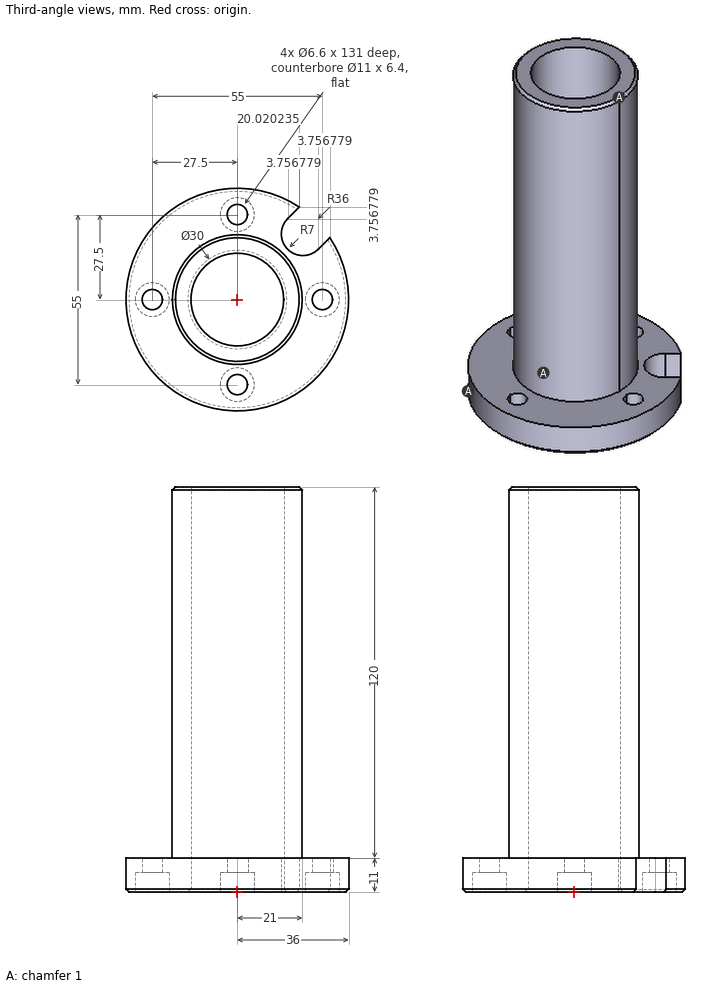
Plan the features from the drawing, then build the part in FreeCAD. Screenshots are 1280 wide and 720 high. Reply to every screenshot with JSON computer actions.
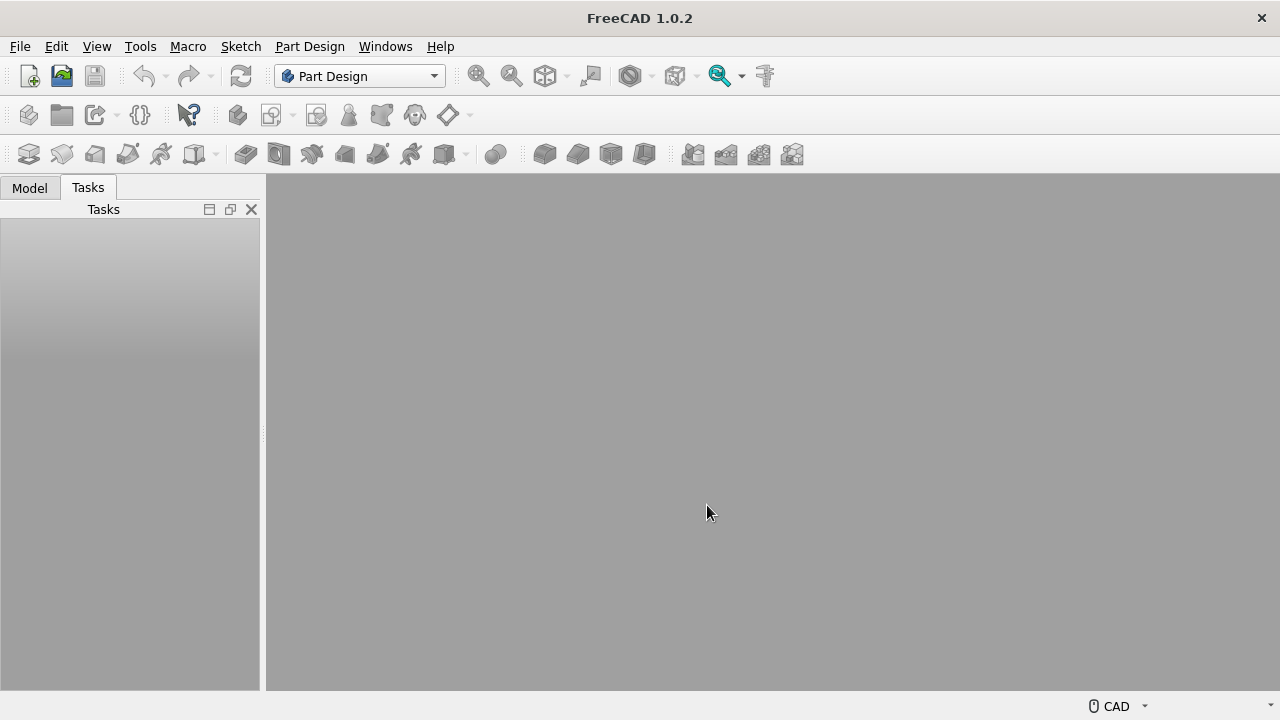
{"action": "left_click", "coordinate": [29, 76]}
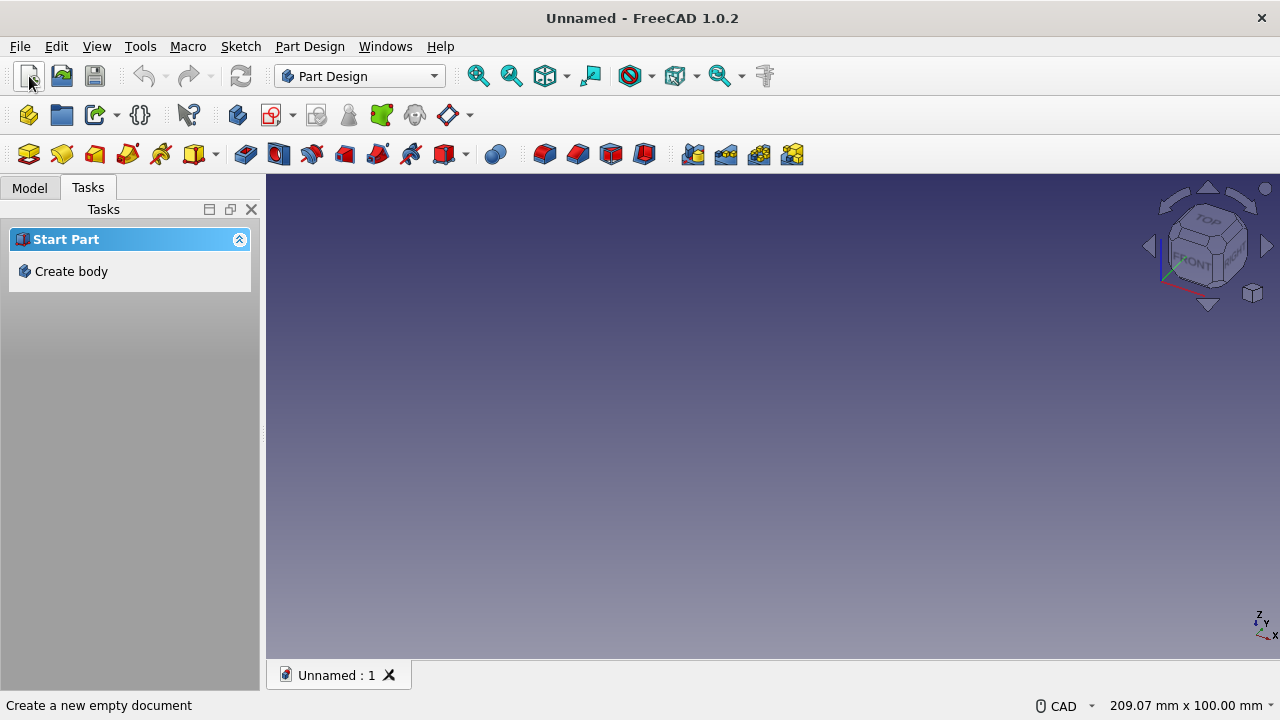
{"action": "left_click", "coordinate": [270, 116]}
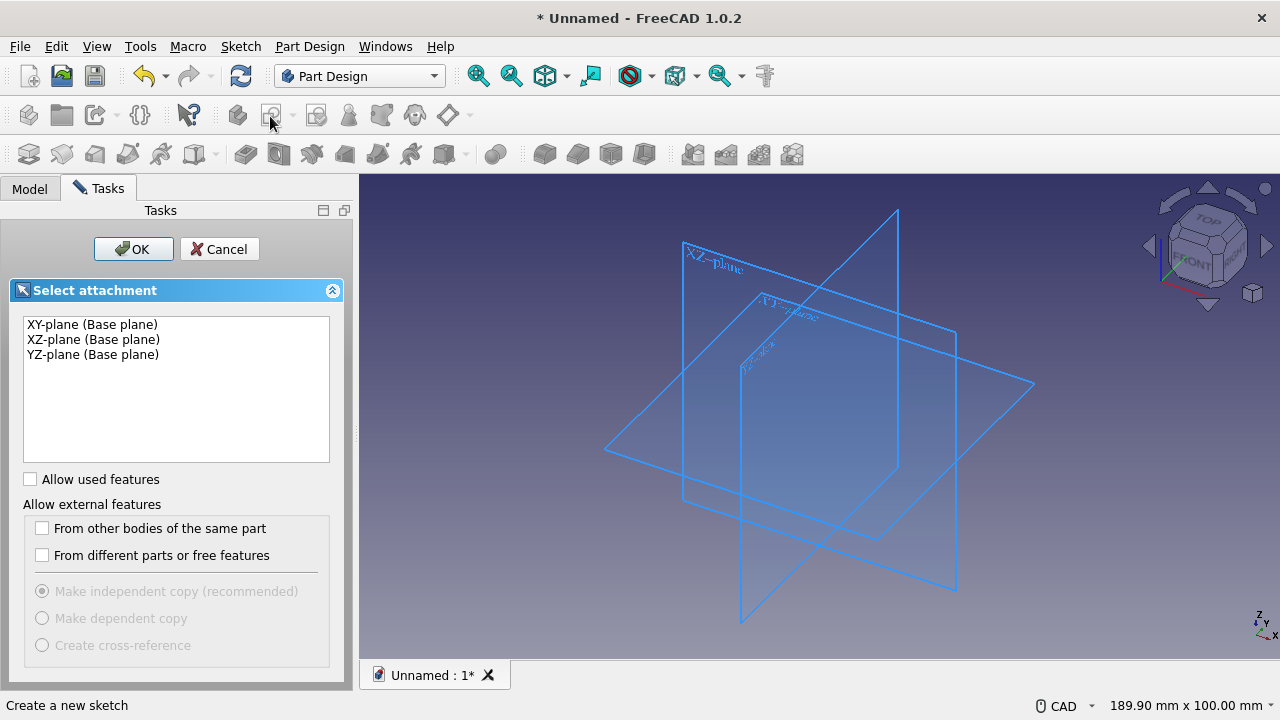
{"action": "left_click", "coordinate": [84, 340]}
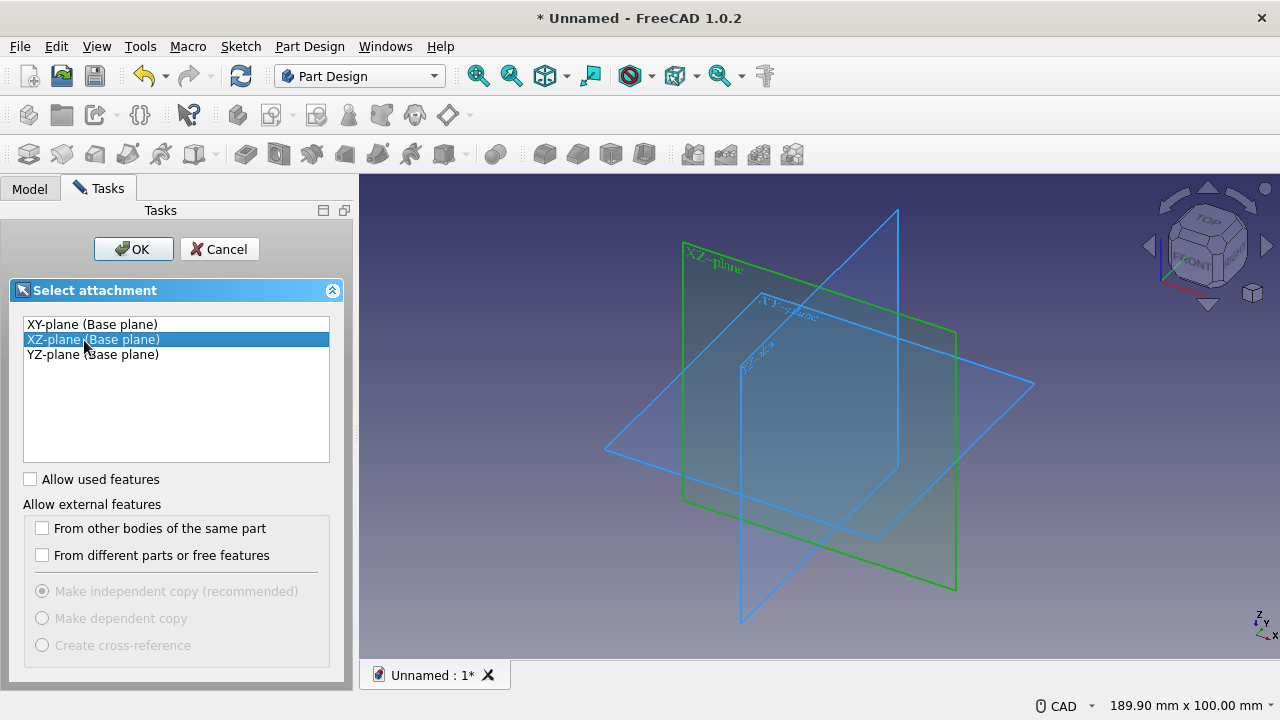
{"action": "left_click", "coordinate": [134, 249]}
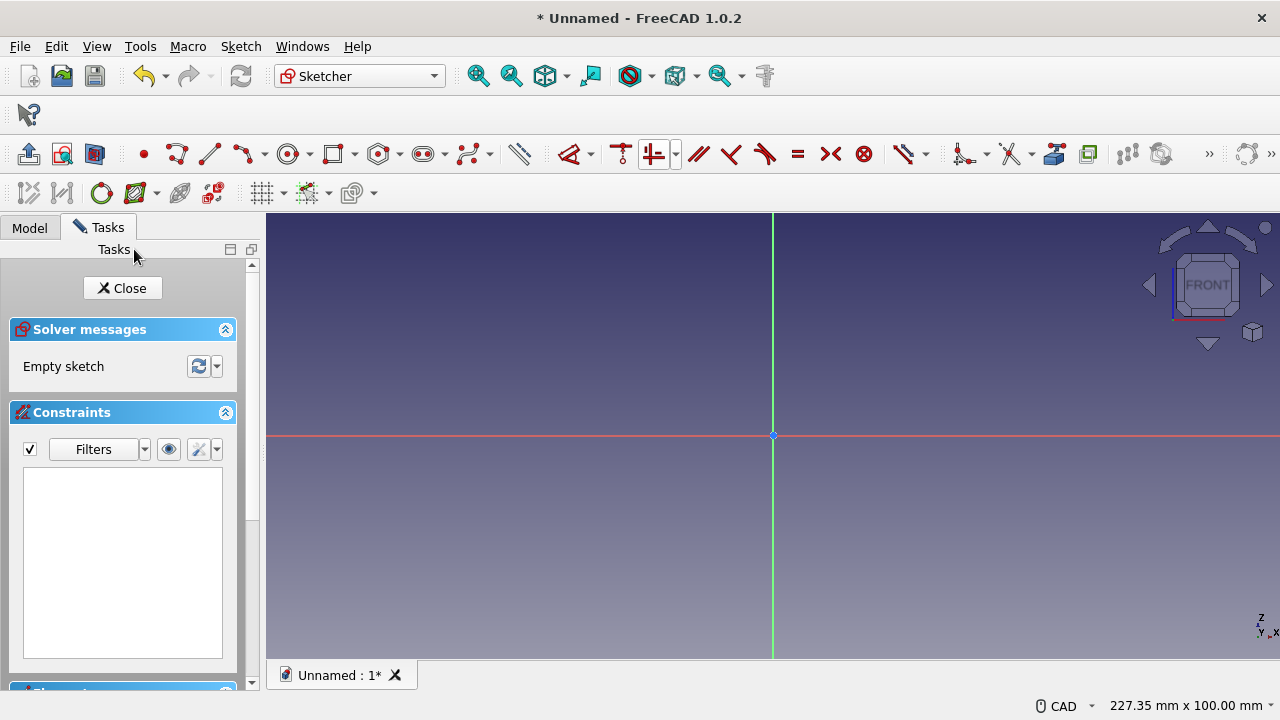
{"action": "scroll", "coordinate": [917, 401], "scroll_direction": "up", "scroll_amount": 6}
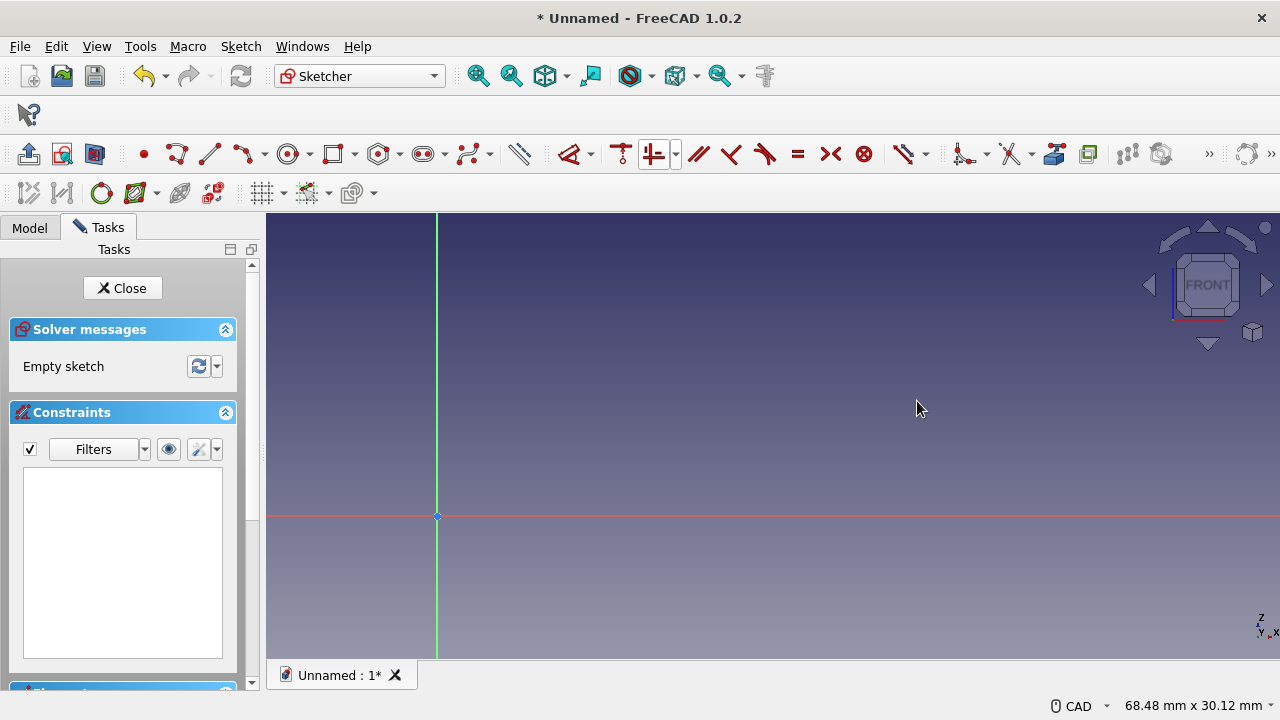
{"action": "left_click", "coordinate": [332, 154]}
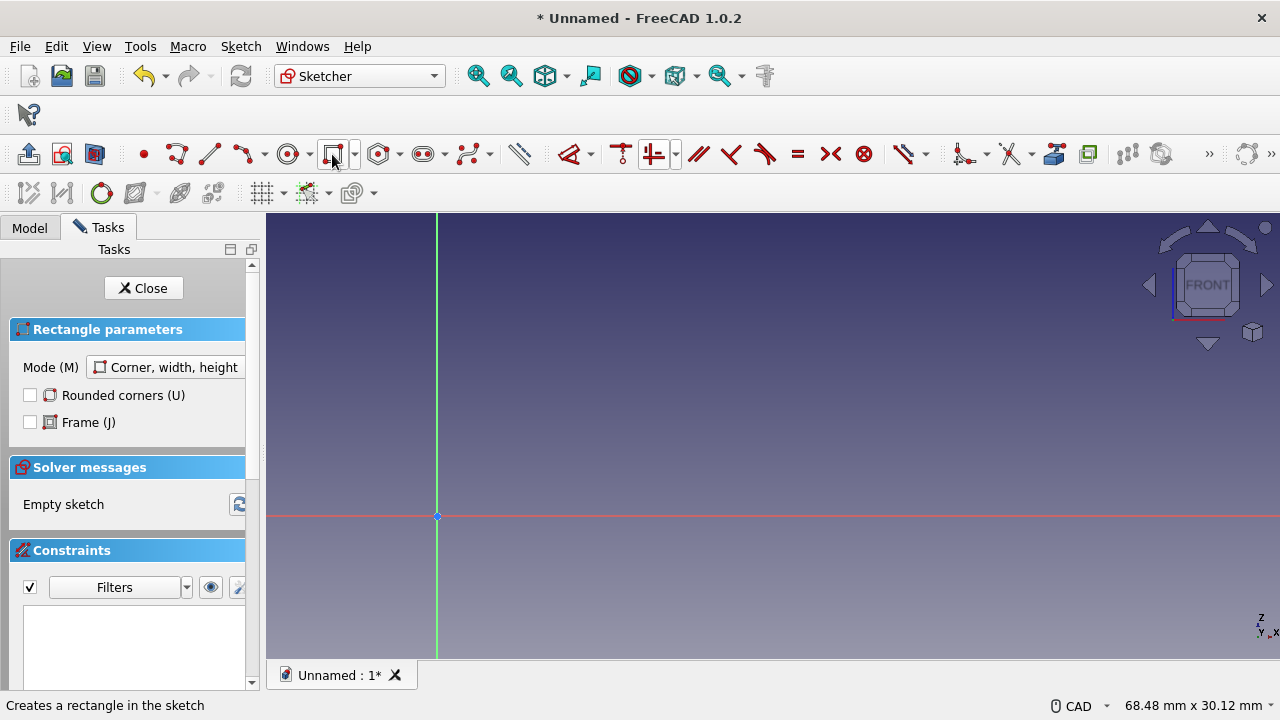
{"action": "left_click", "coordinate": [437, 516]}
{"action": "mouse_move", "coordinate": [970, 353]}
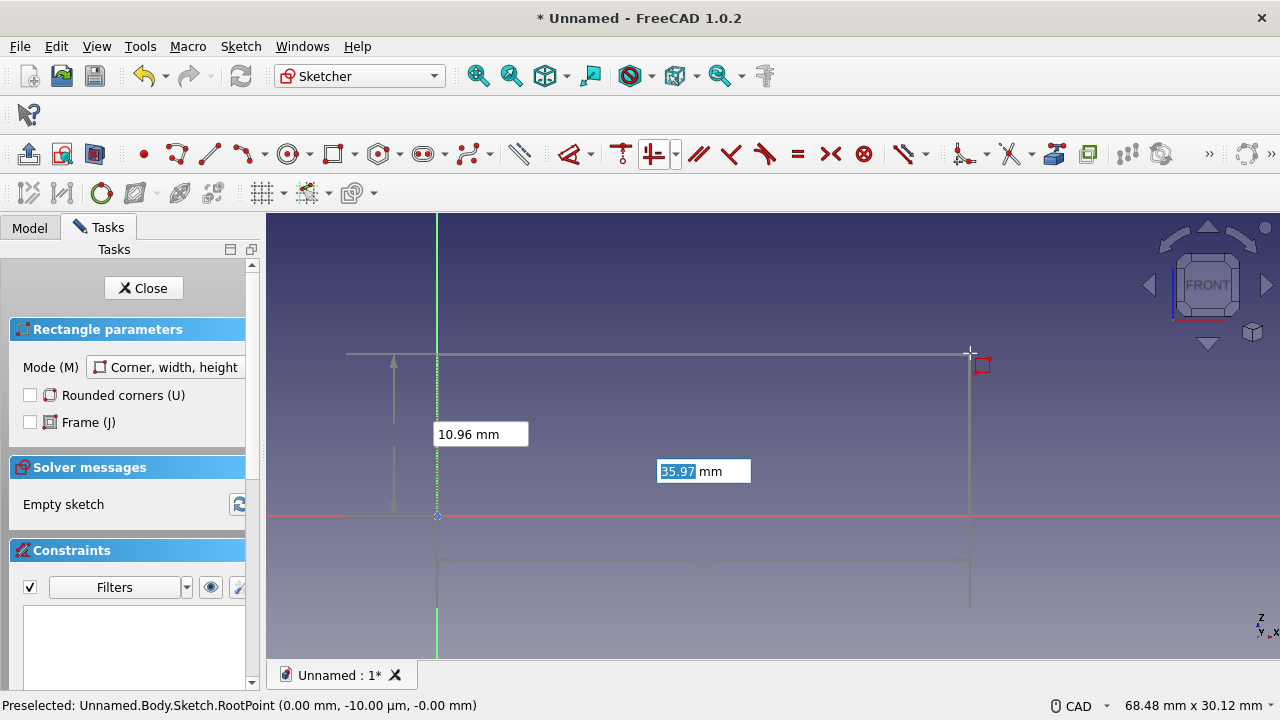
{"action": "type", "text": "36"}
{"action": "key", "text": "Tab"}
{"action": "type", "text": "11"}
{"action": "key", "text": "Return"}
{"action": "key", "text": "Escape"}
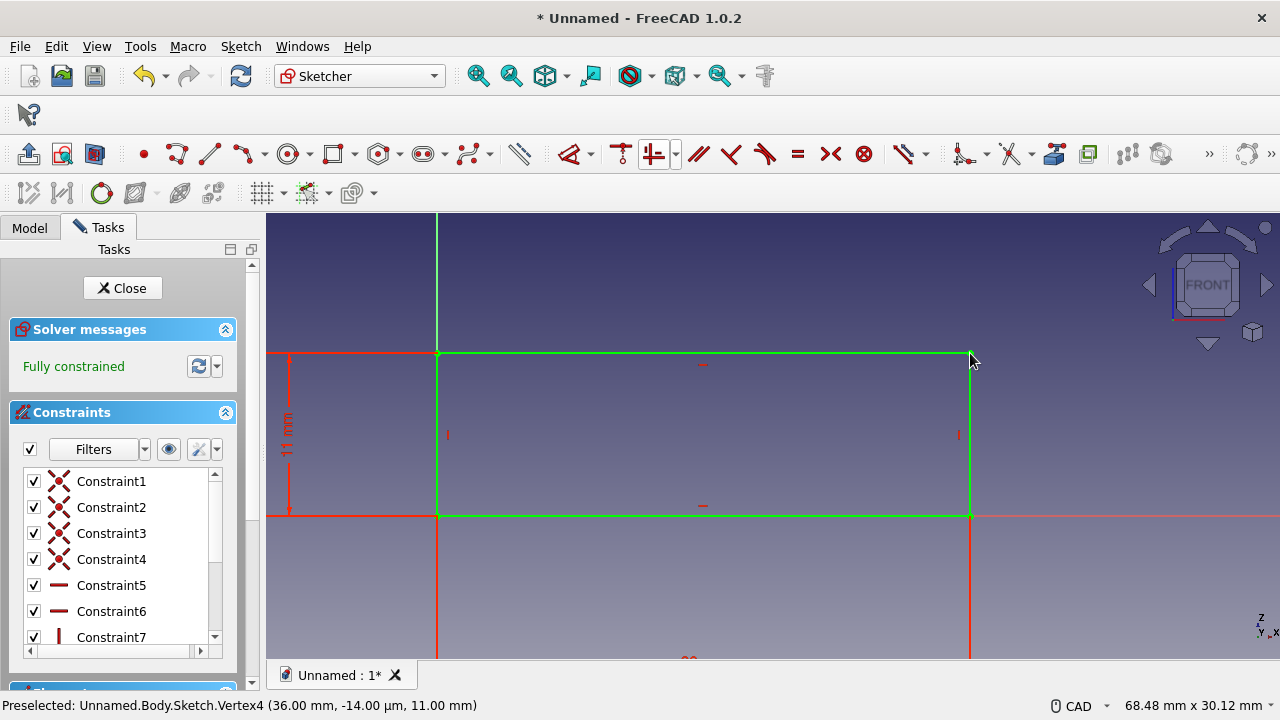
{"action": "left_click", "coordinate": [123, 288]}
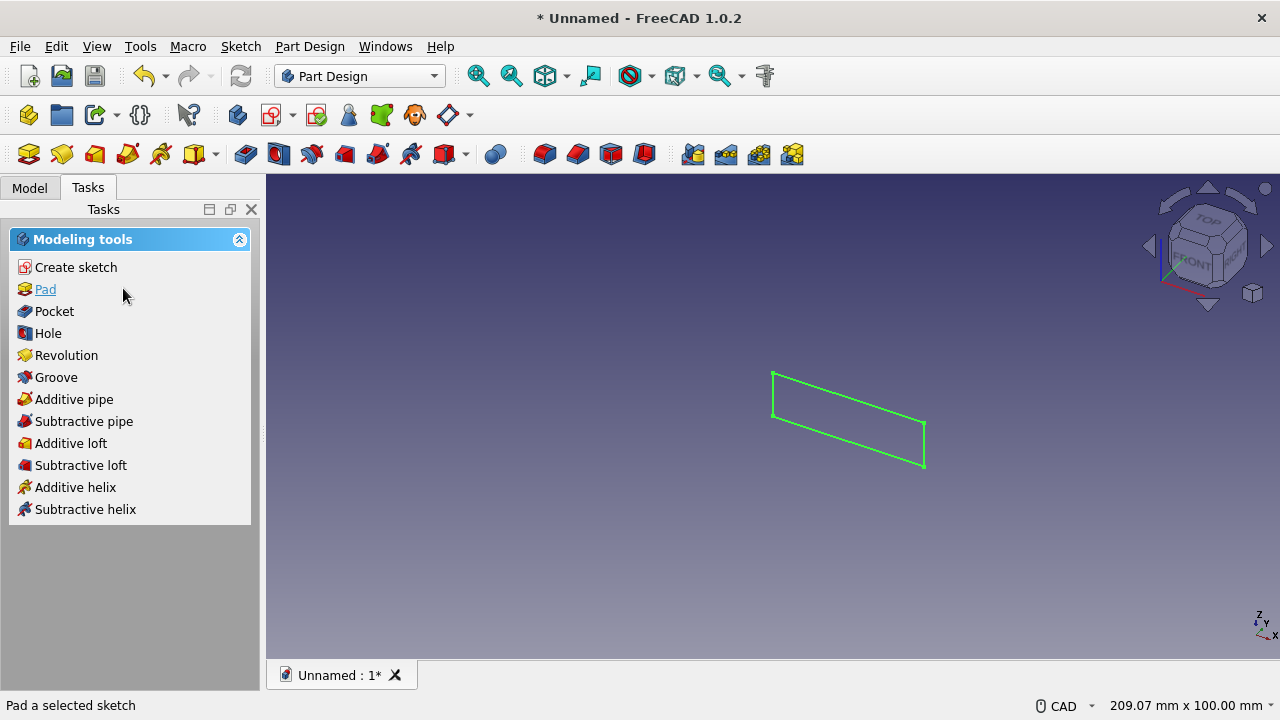
{"action": "left_click", "coordinate": [62, 154]}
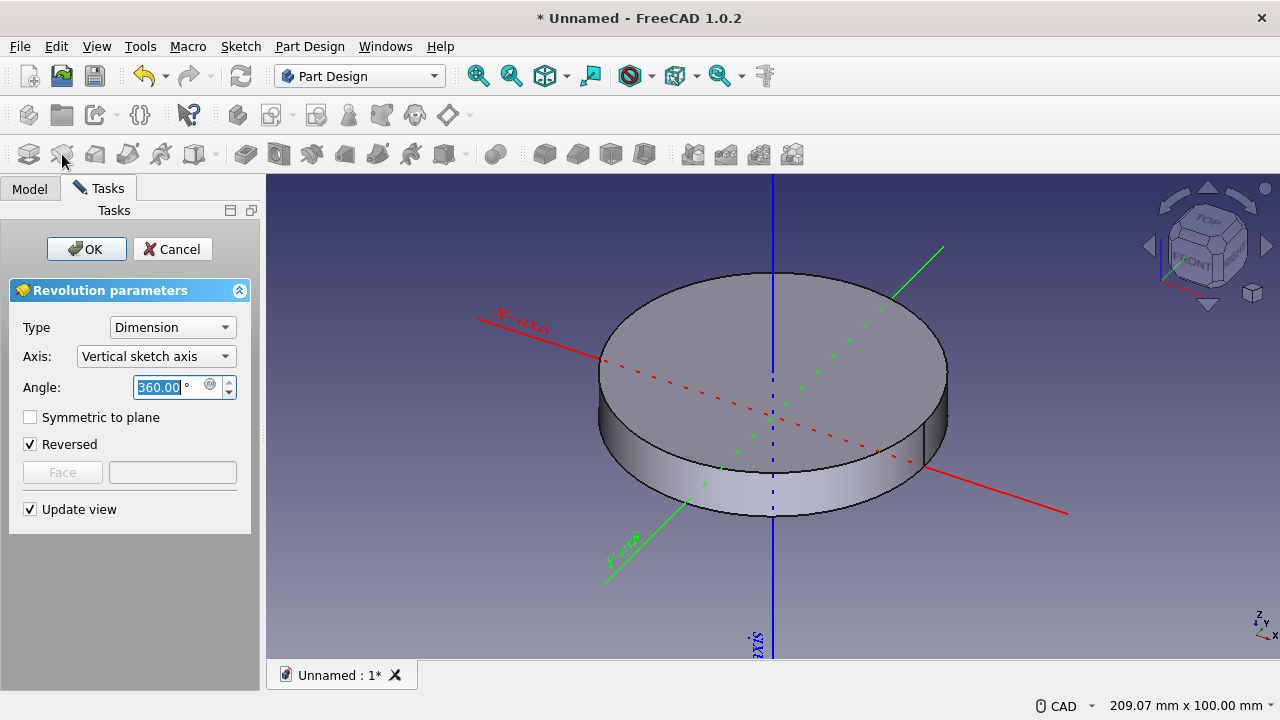
{"action": "left_click", "coordinate": [87, 249]}